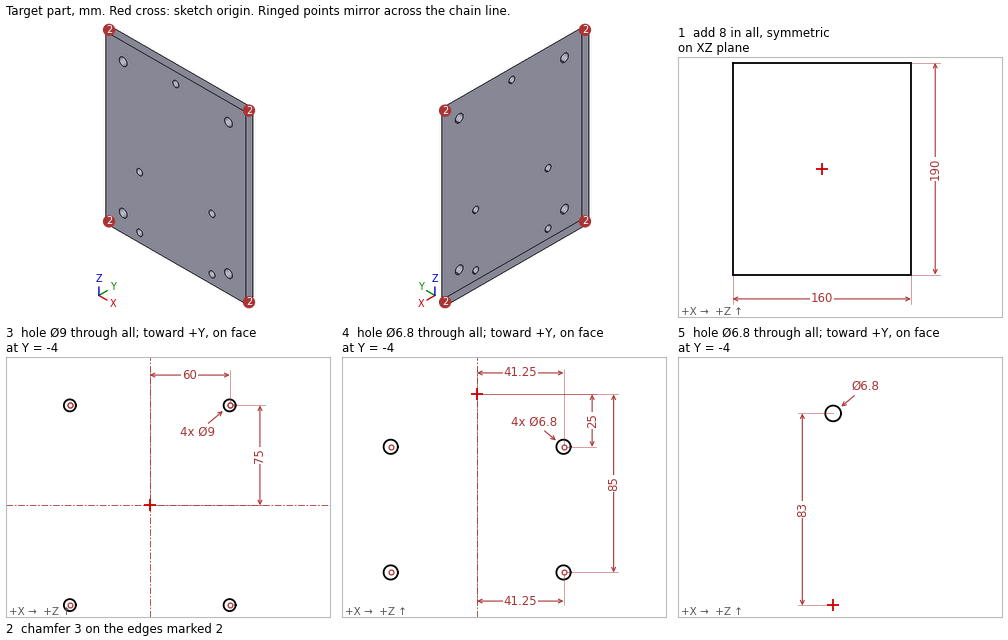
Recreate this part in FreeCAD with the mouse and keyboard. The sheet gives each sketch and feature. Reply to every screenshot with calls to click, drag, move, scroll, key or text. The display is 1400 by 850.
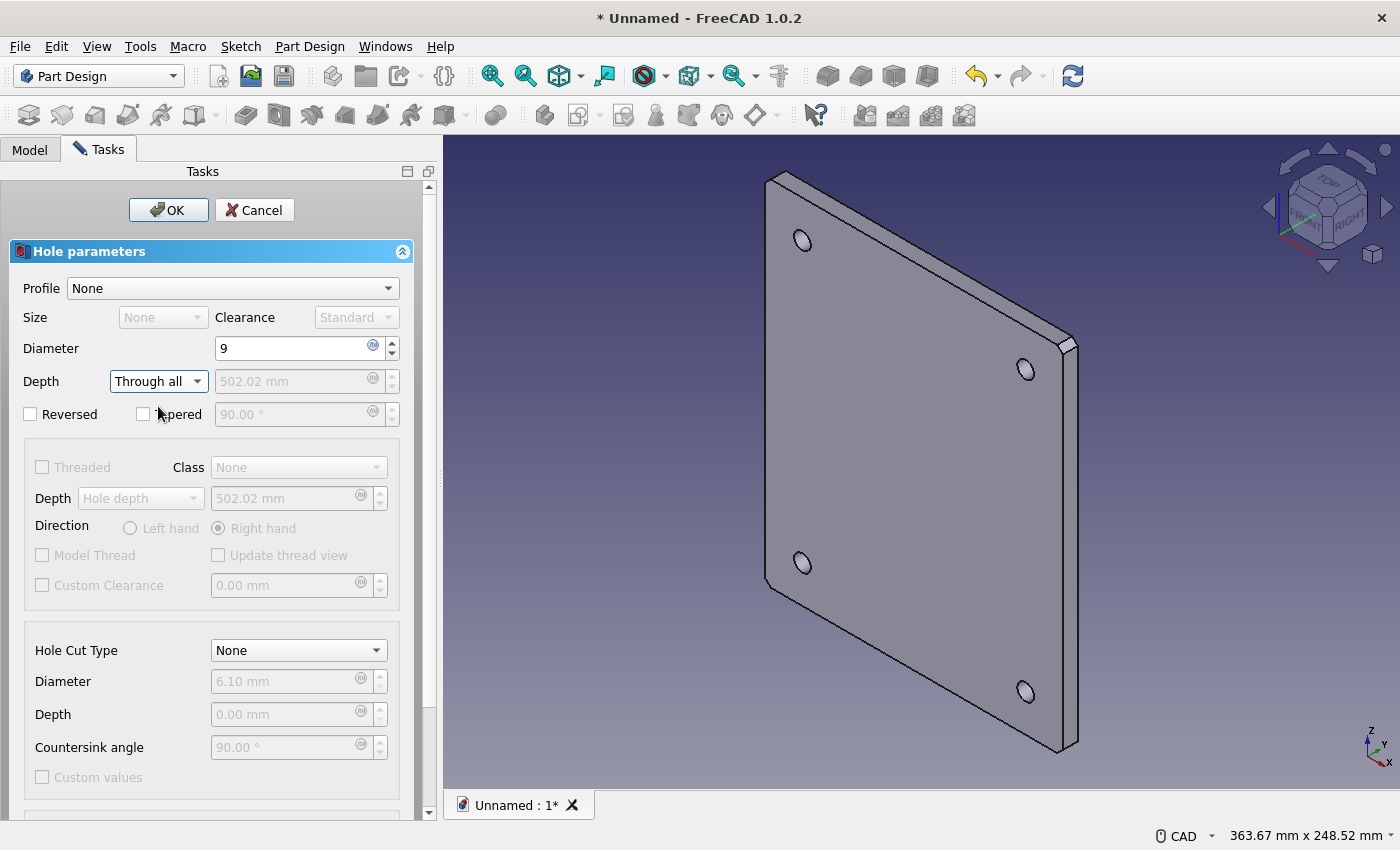
click(169, 210)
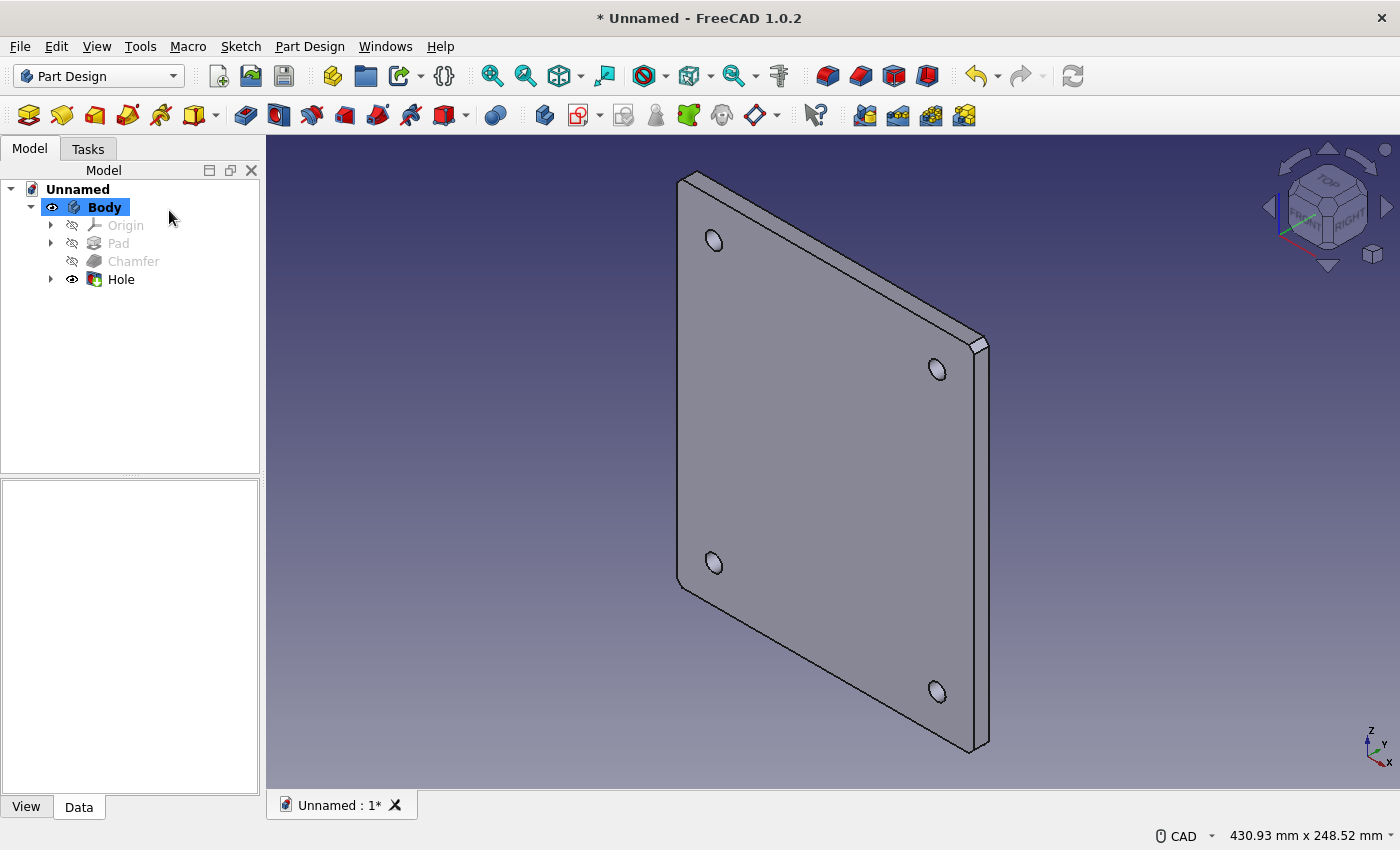
click(826, 465)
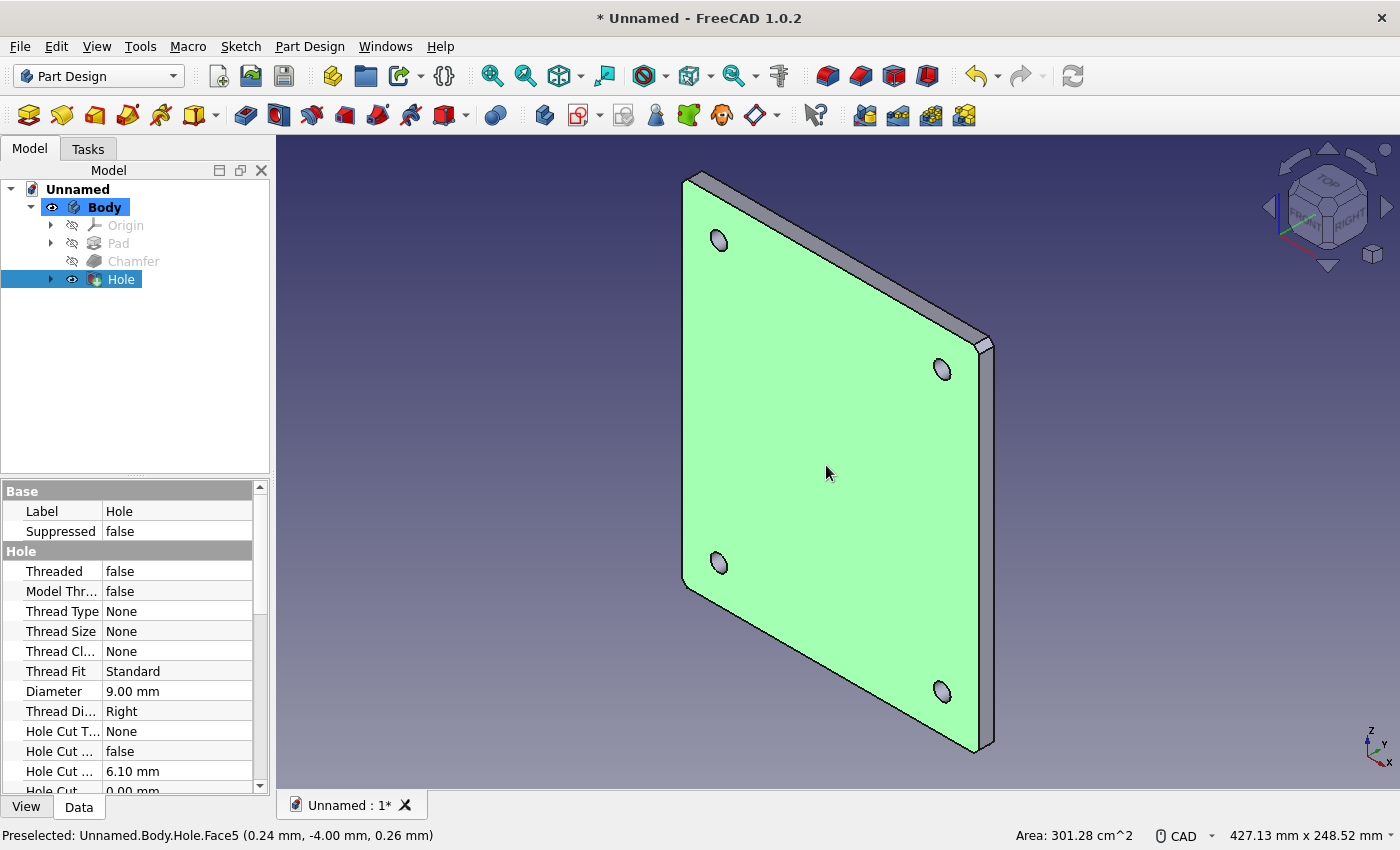
click(578, 116)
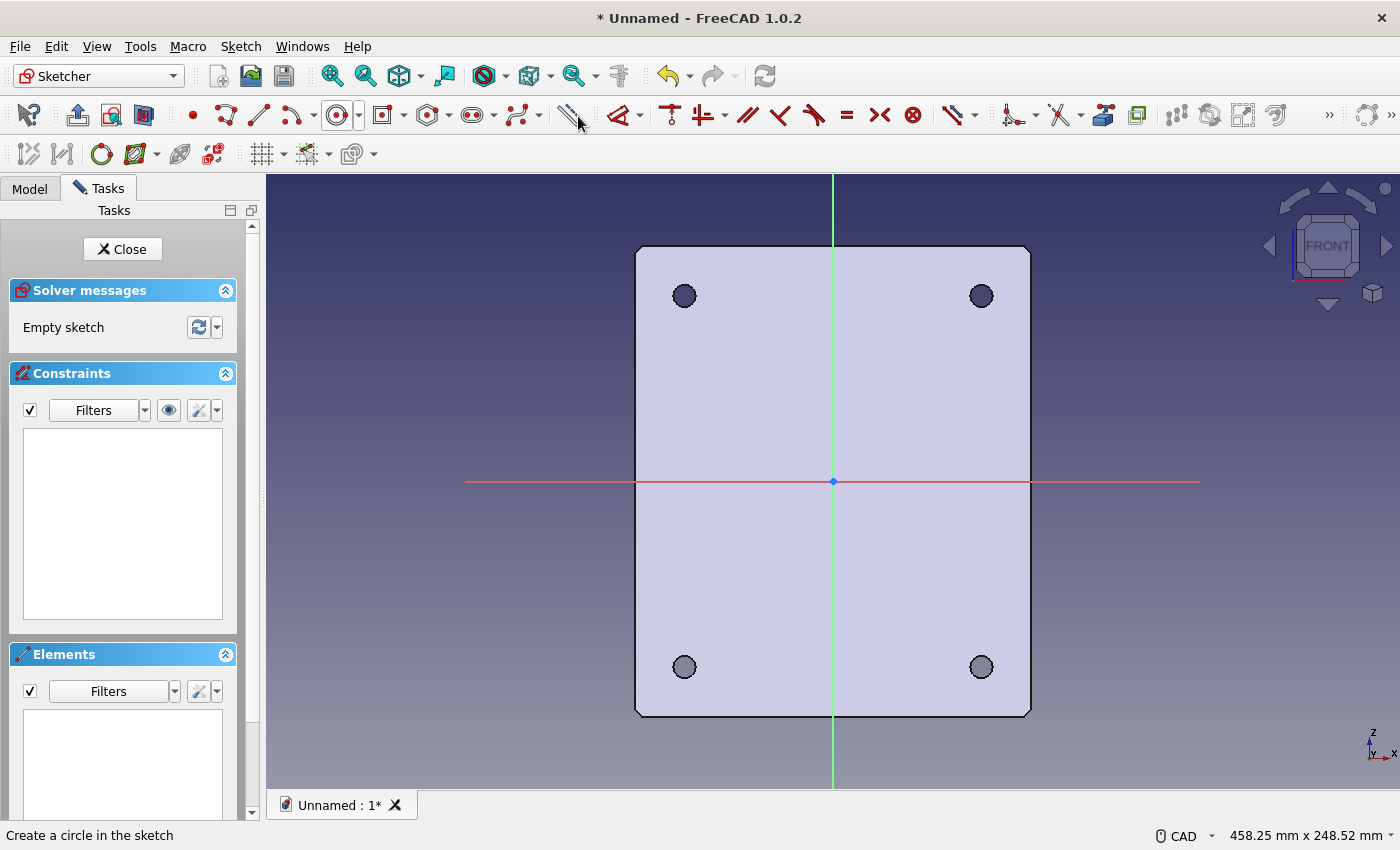
scroll(916, 724, up, 3)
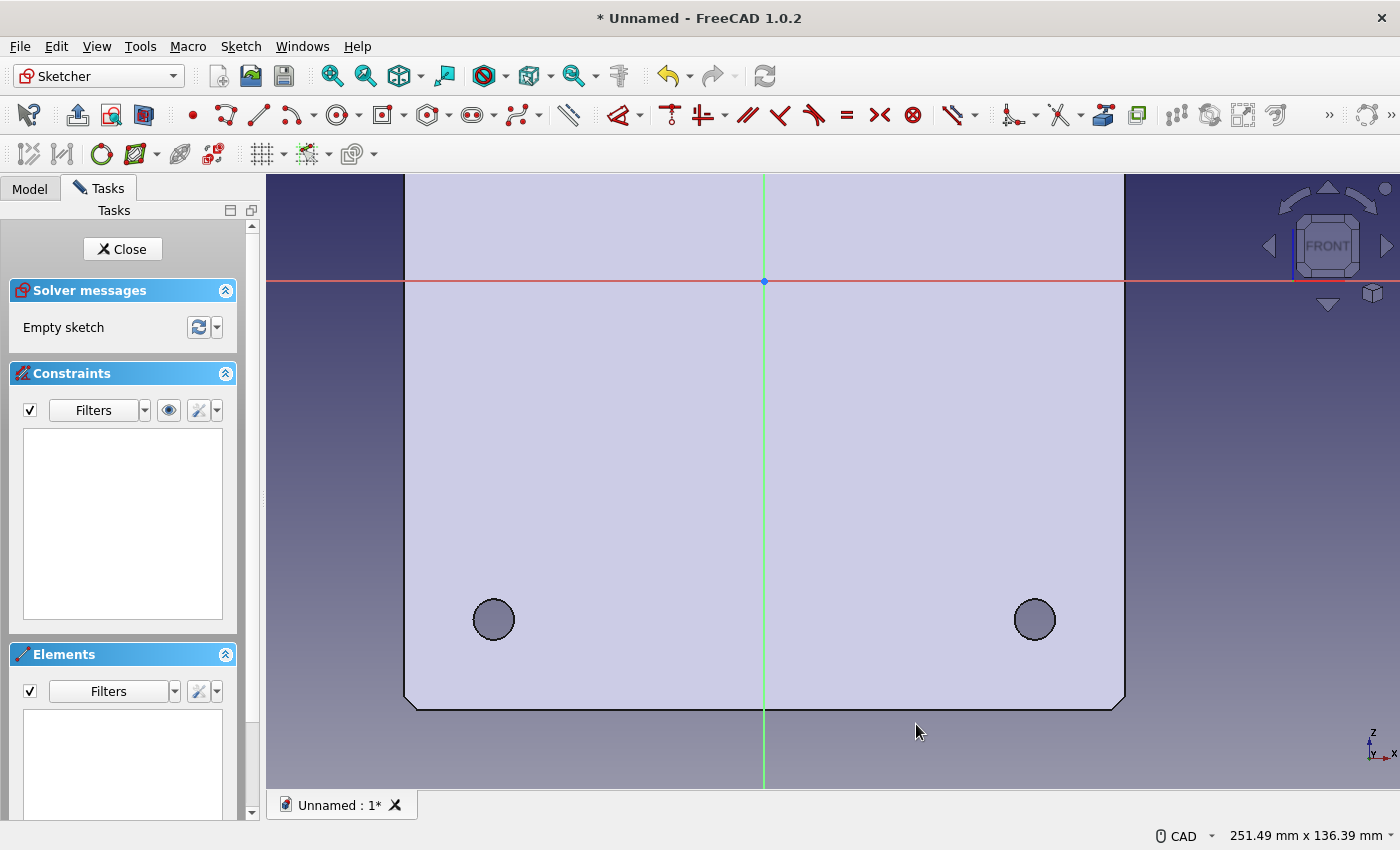
click(336, 116)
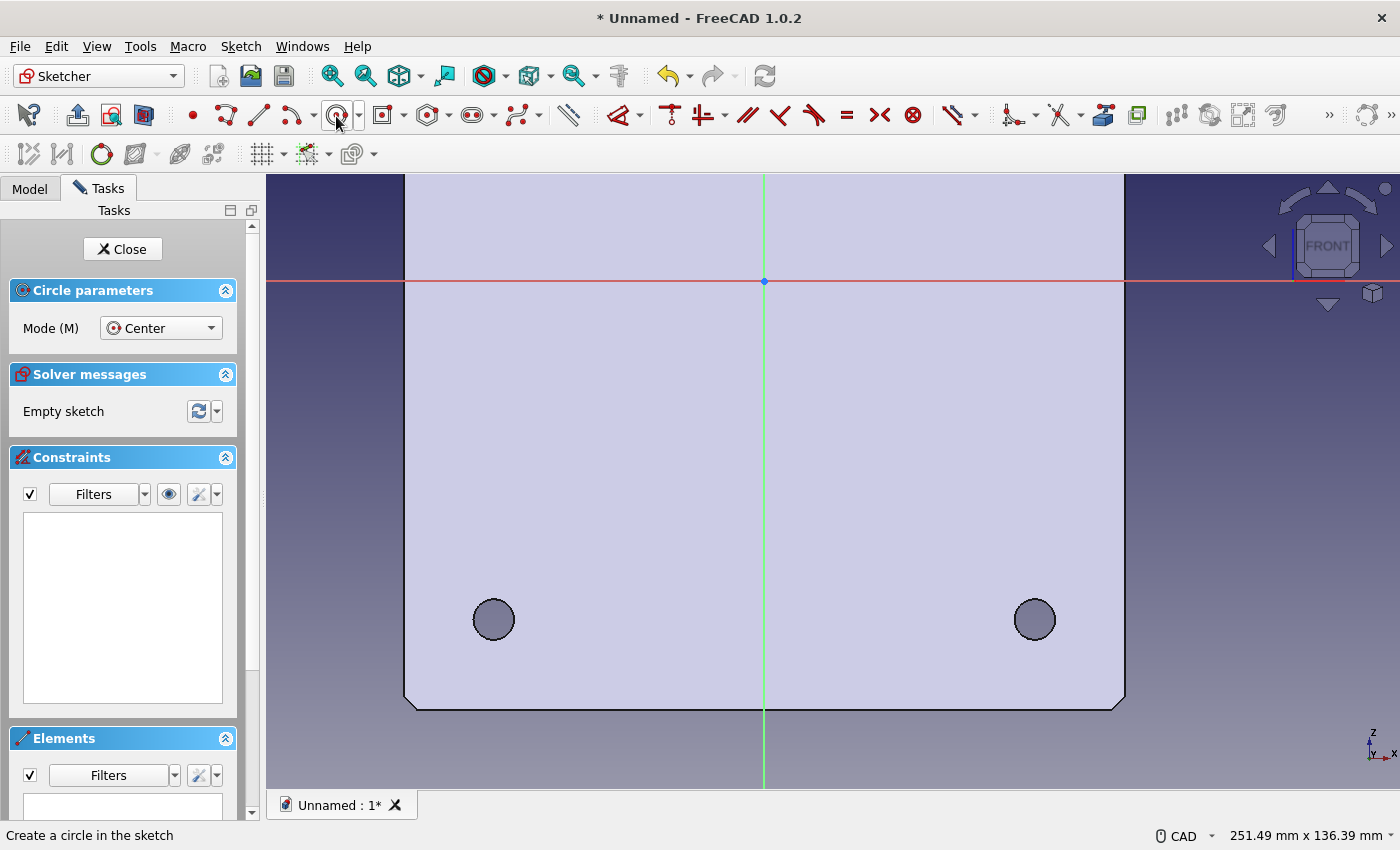
scroll(950, 394, up, 2)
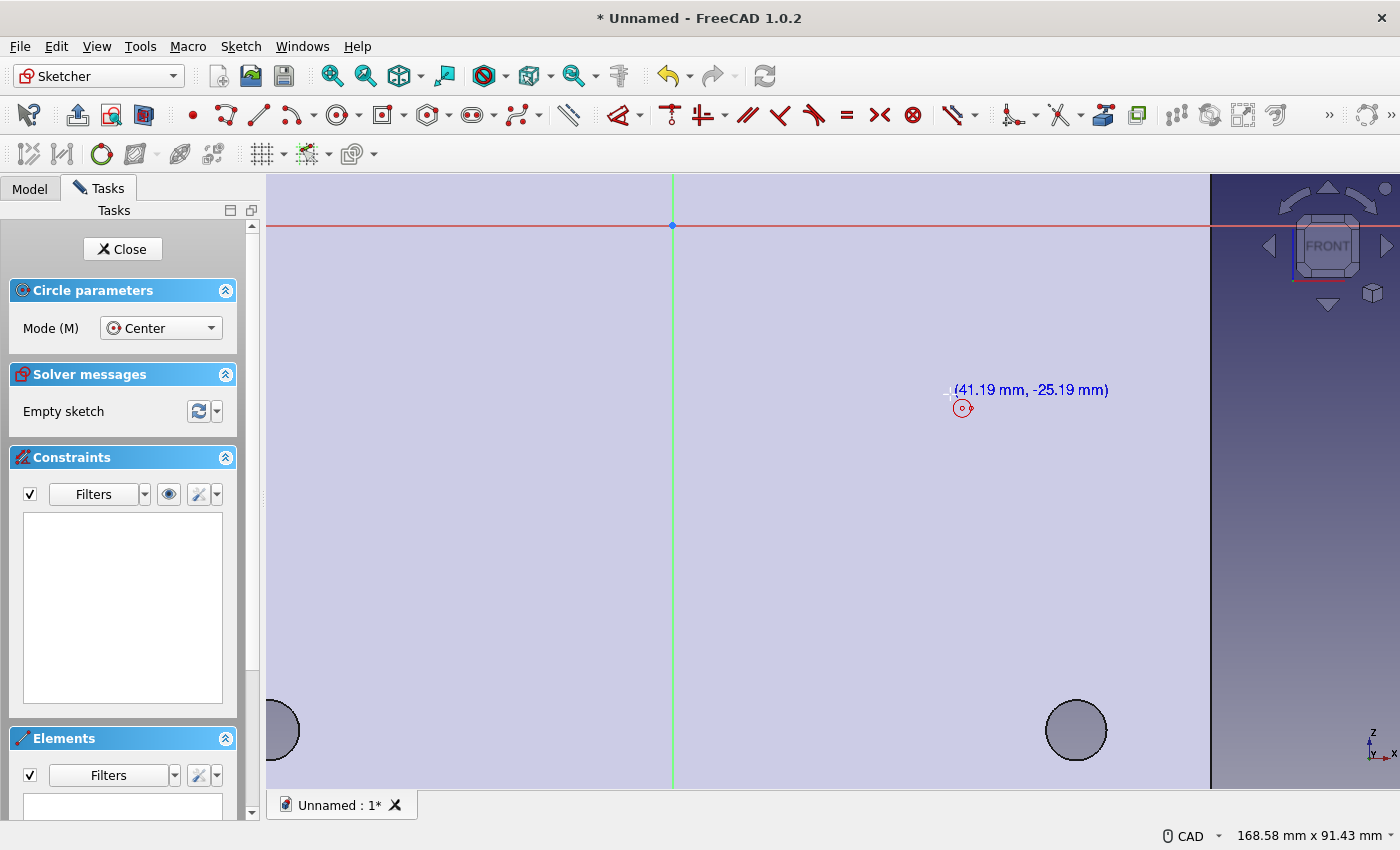
click(950, 394)
click(966, 378)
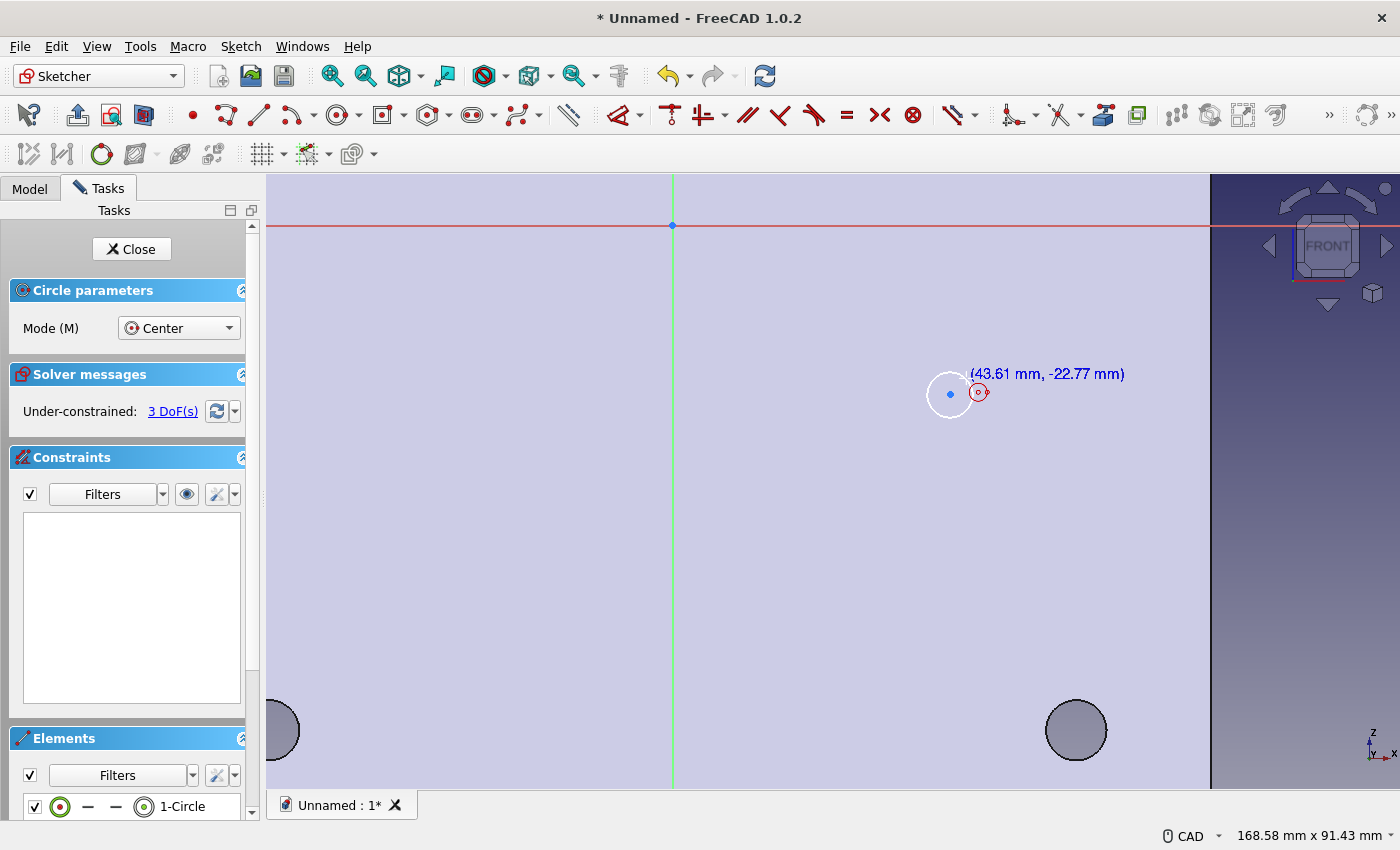
scroll(951, 397, down, 2)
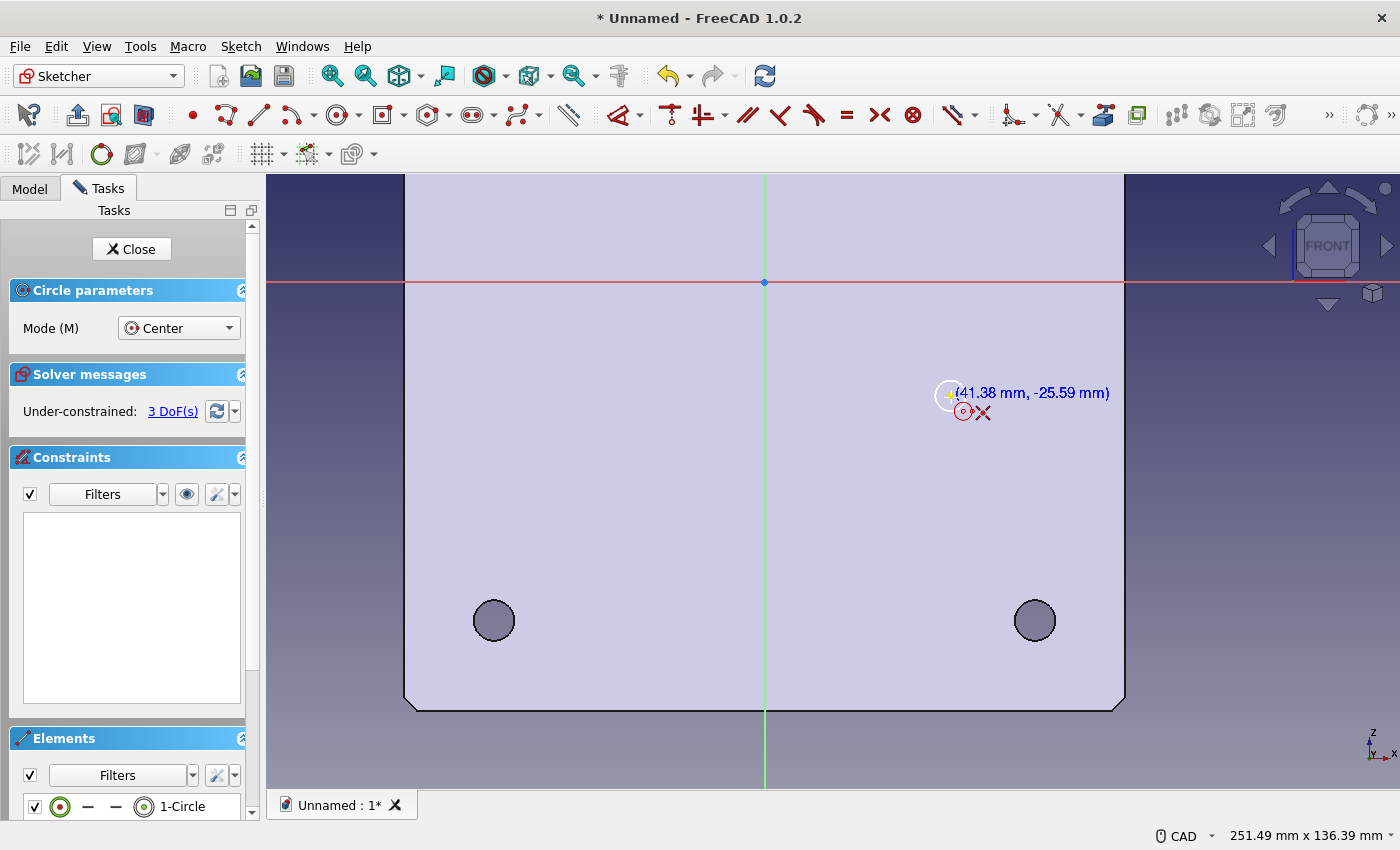
scroll(951, 666, up, 2)